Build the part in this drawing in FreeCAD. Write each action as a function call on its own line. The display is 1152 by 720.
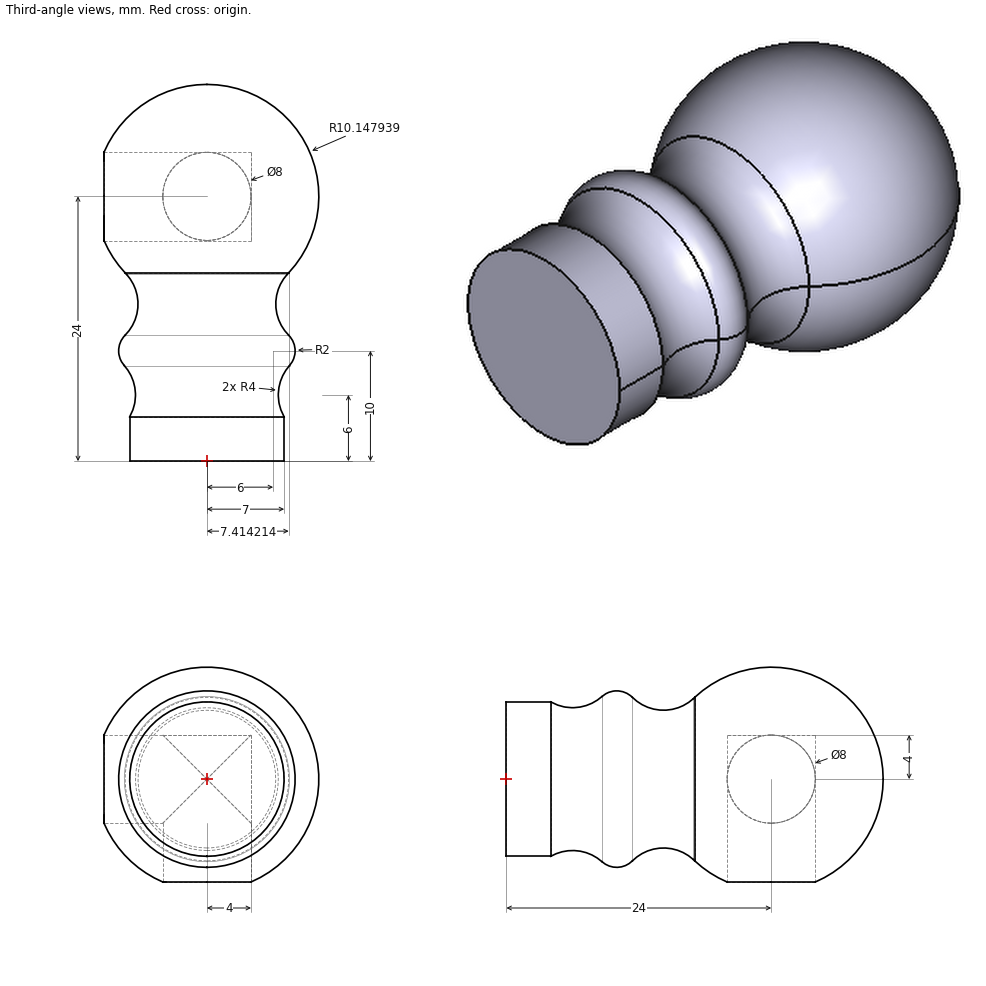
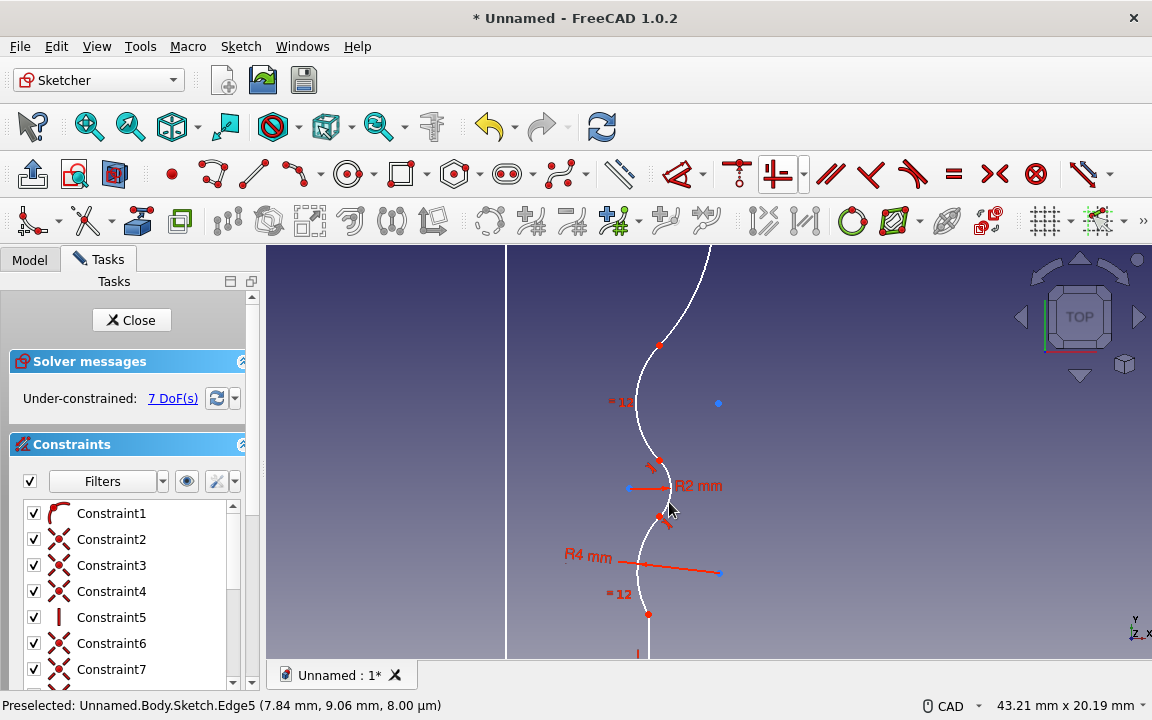
scroll(663, 515, down, 5)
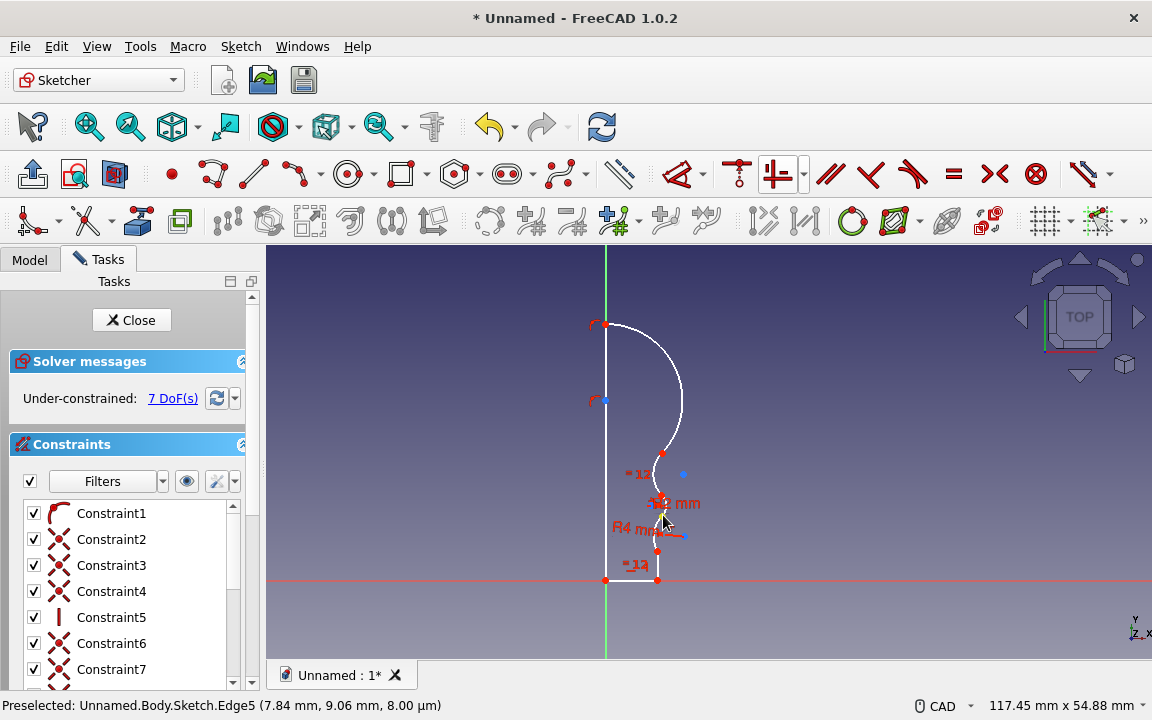
click(682, 405)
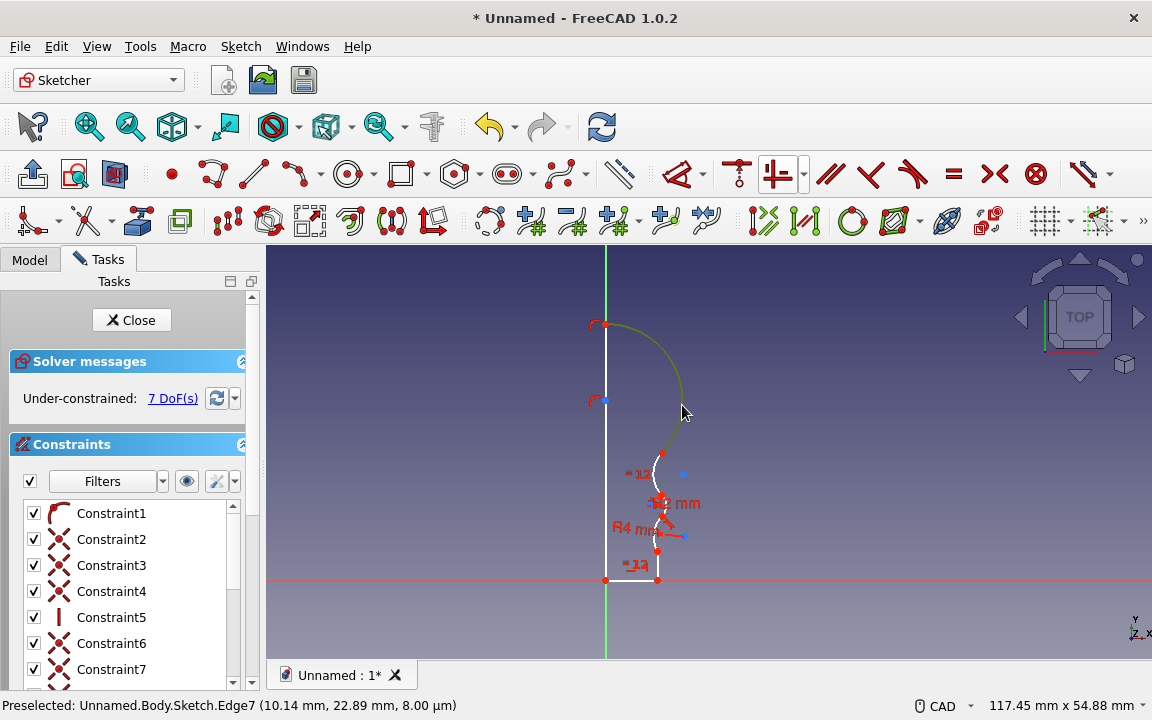
key(k)
key(r)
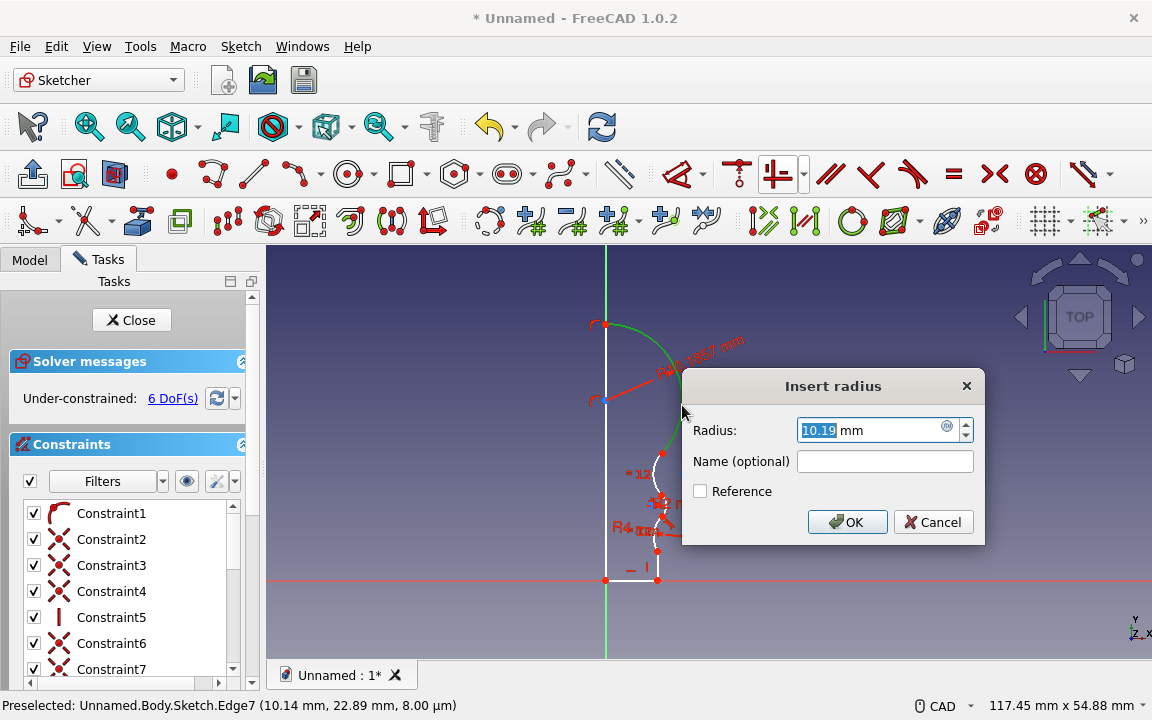
text(10.147939)
key(Return)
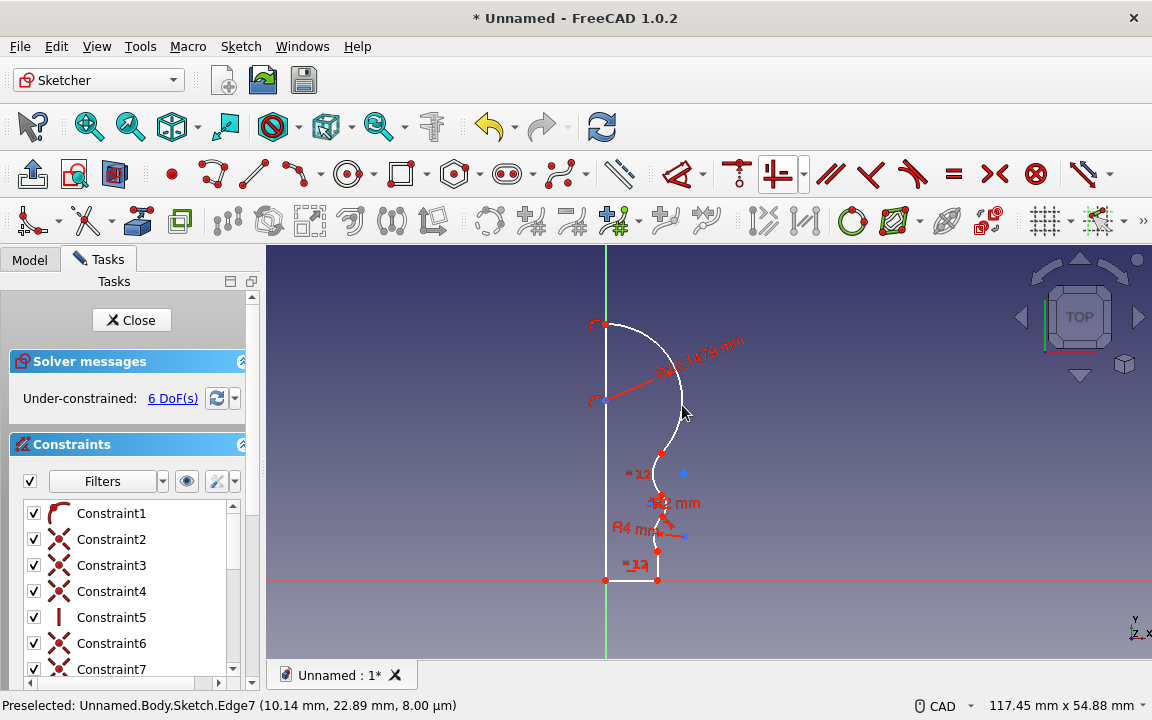
click(621, 581)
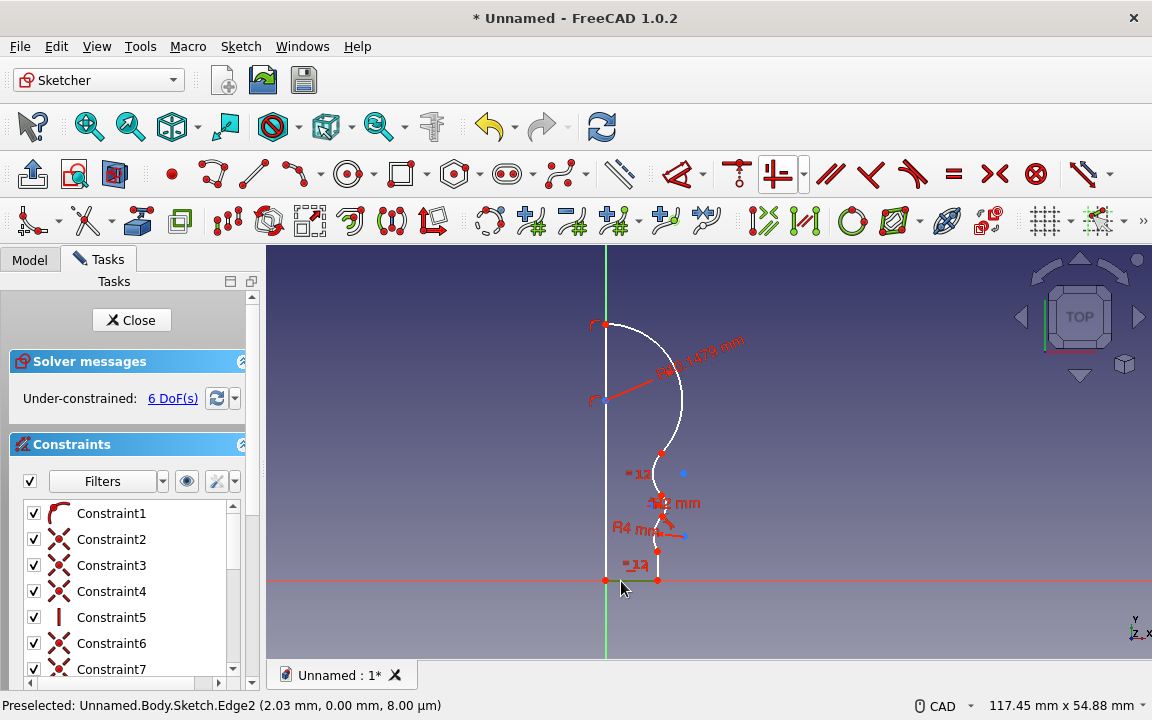
click(702, 174)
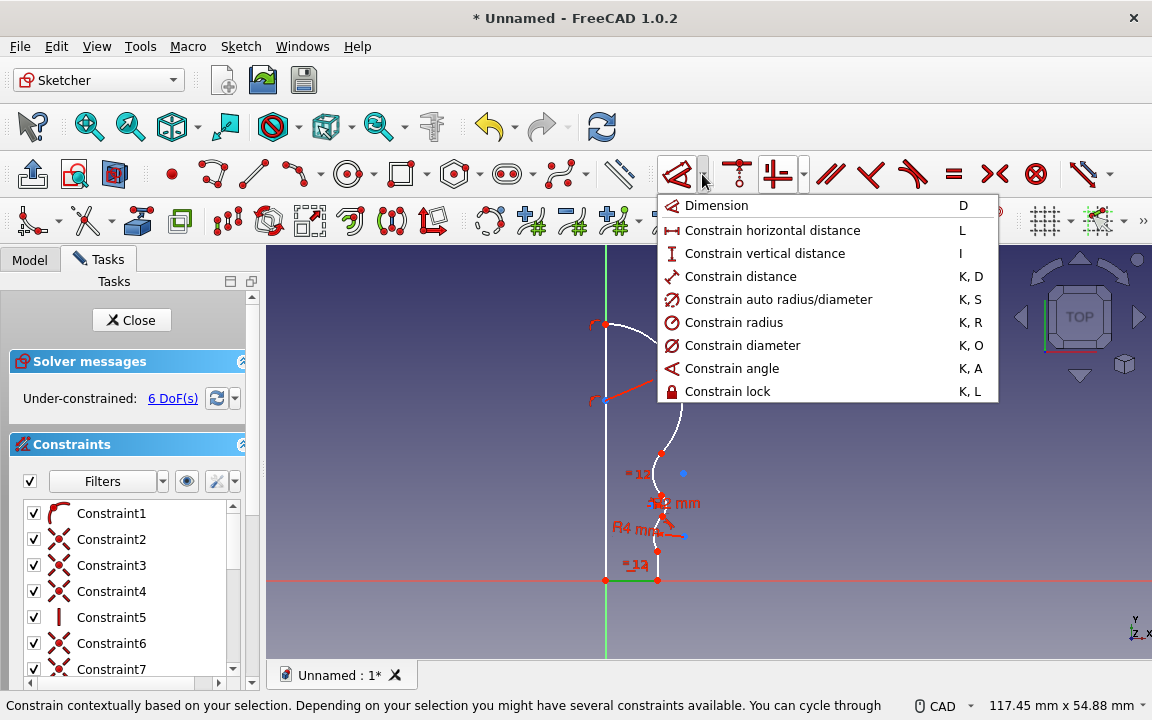
click(828, 230)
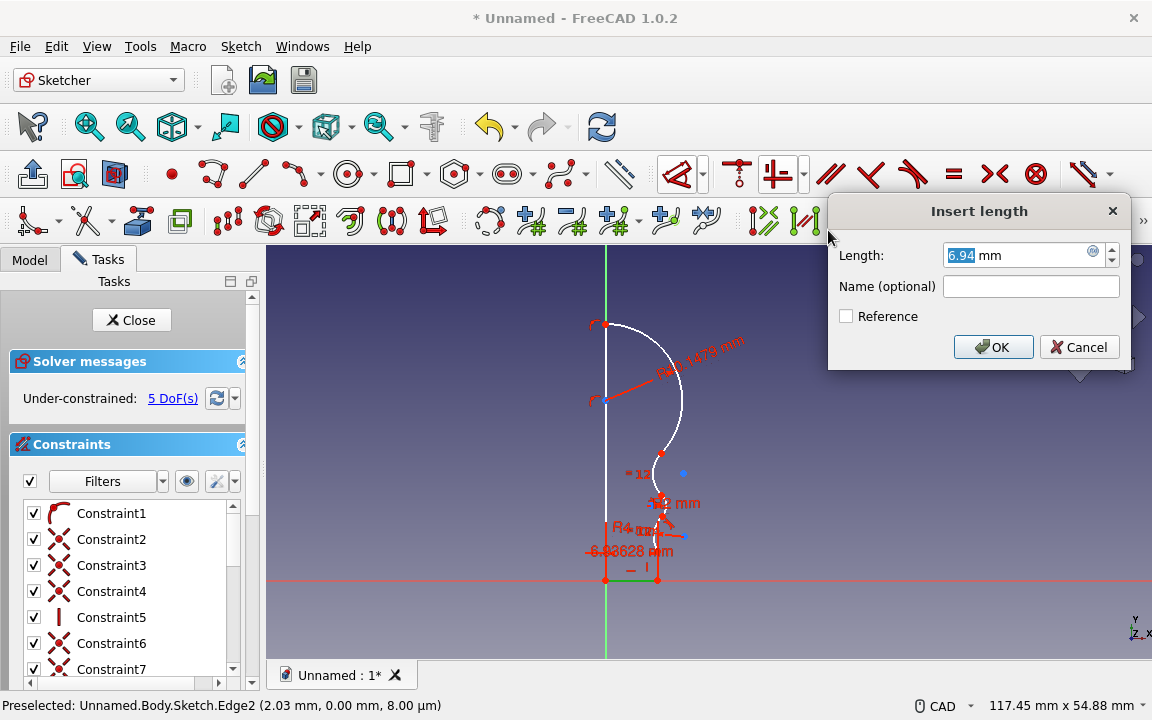
text(7)
key(Return)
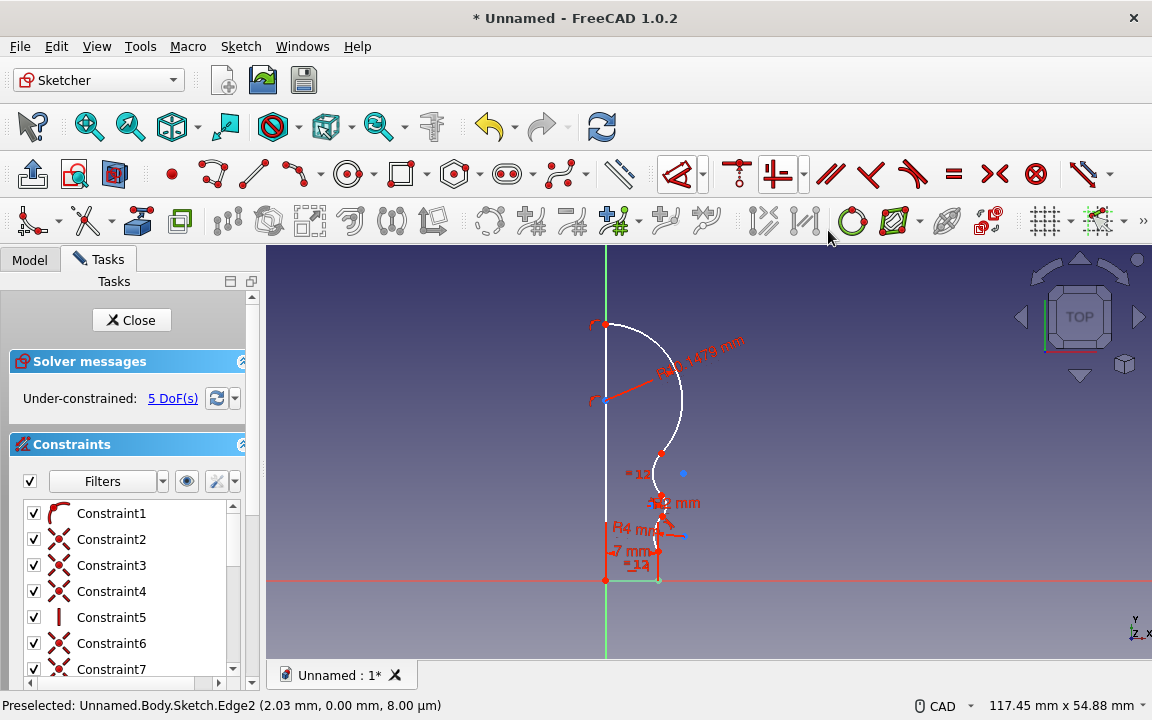
click(684, 537)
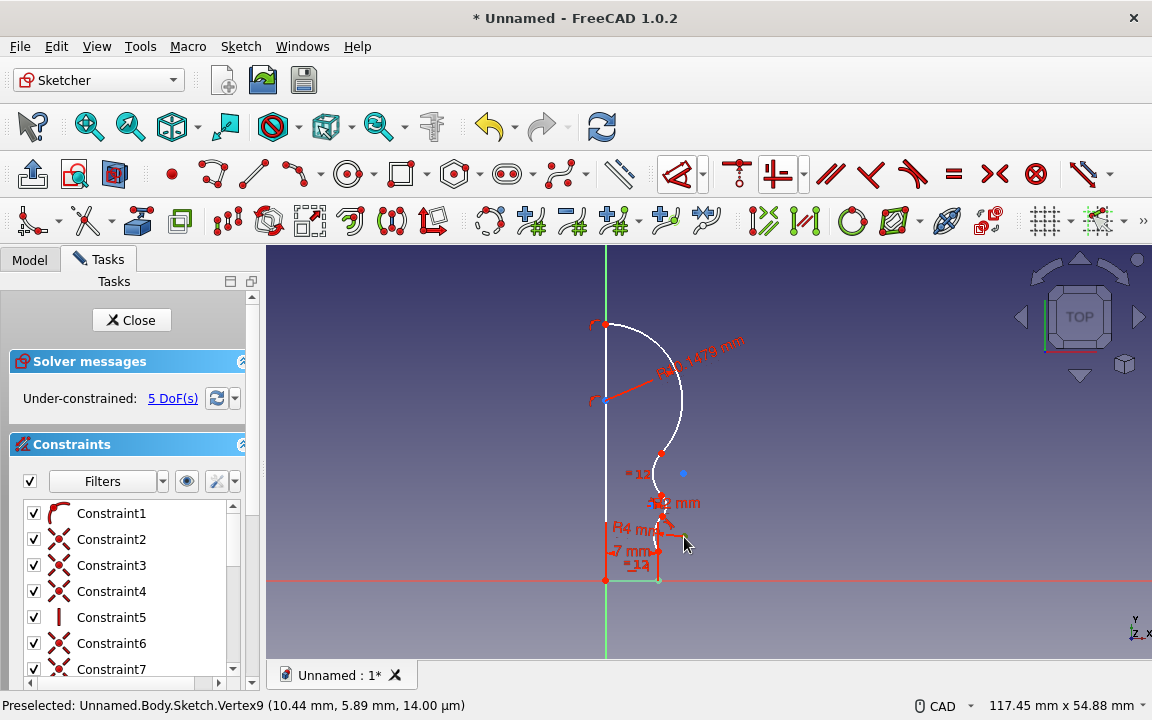
click(702, 174)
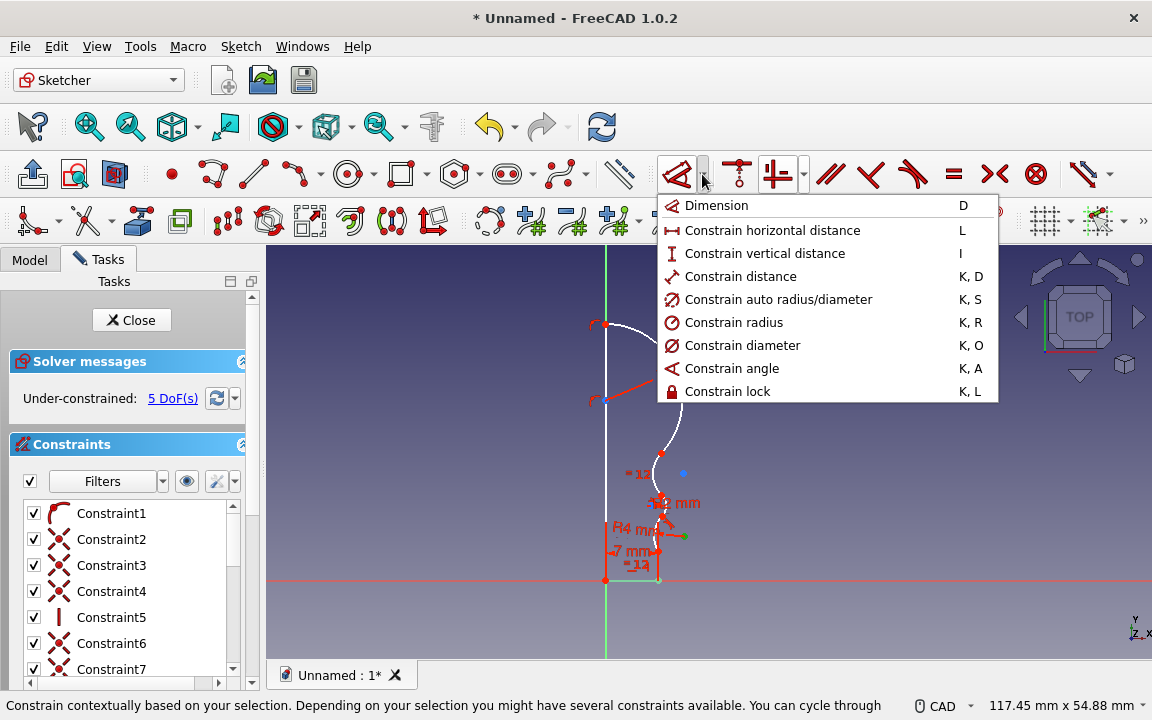
click(828, 254)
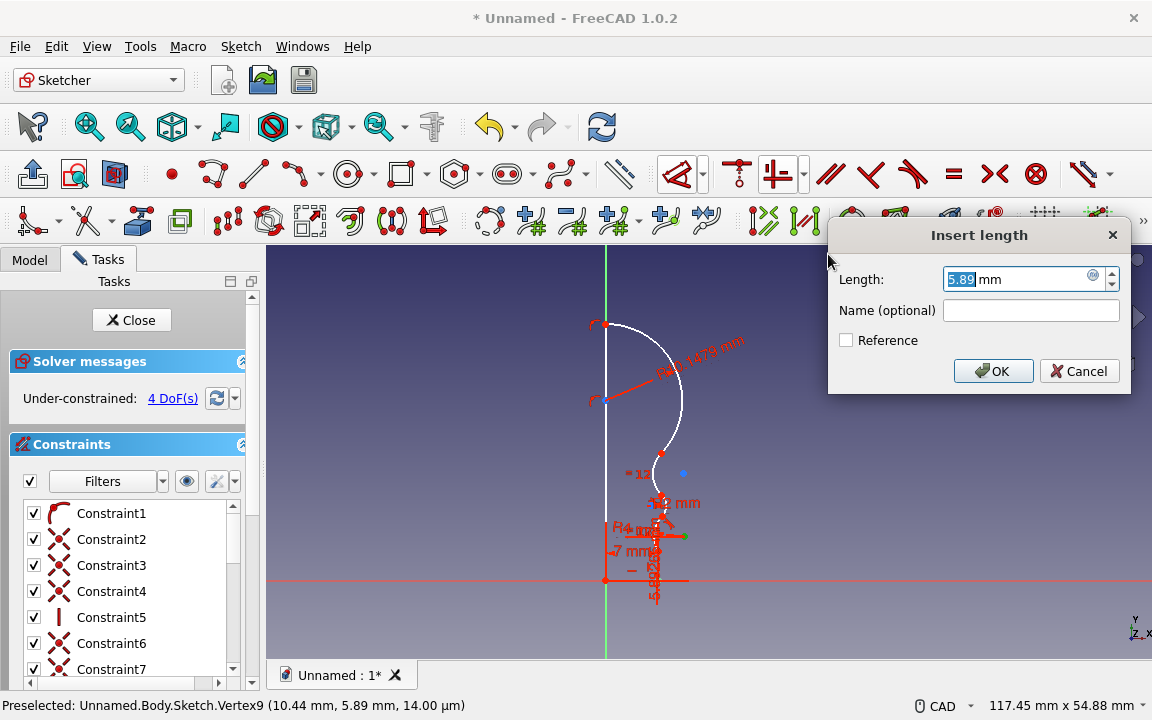
text(6)
key(Return)